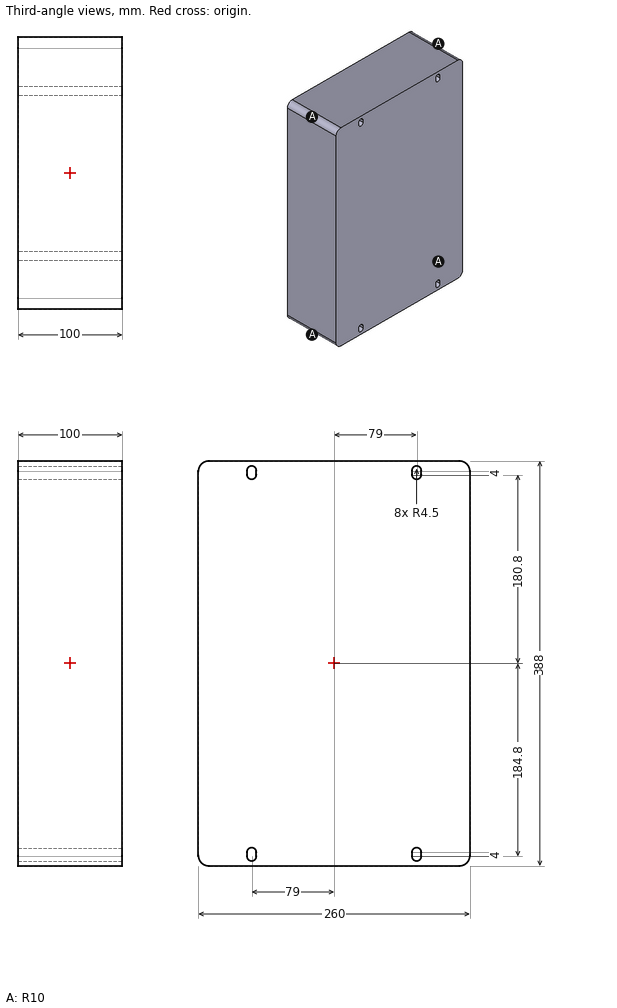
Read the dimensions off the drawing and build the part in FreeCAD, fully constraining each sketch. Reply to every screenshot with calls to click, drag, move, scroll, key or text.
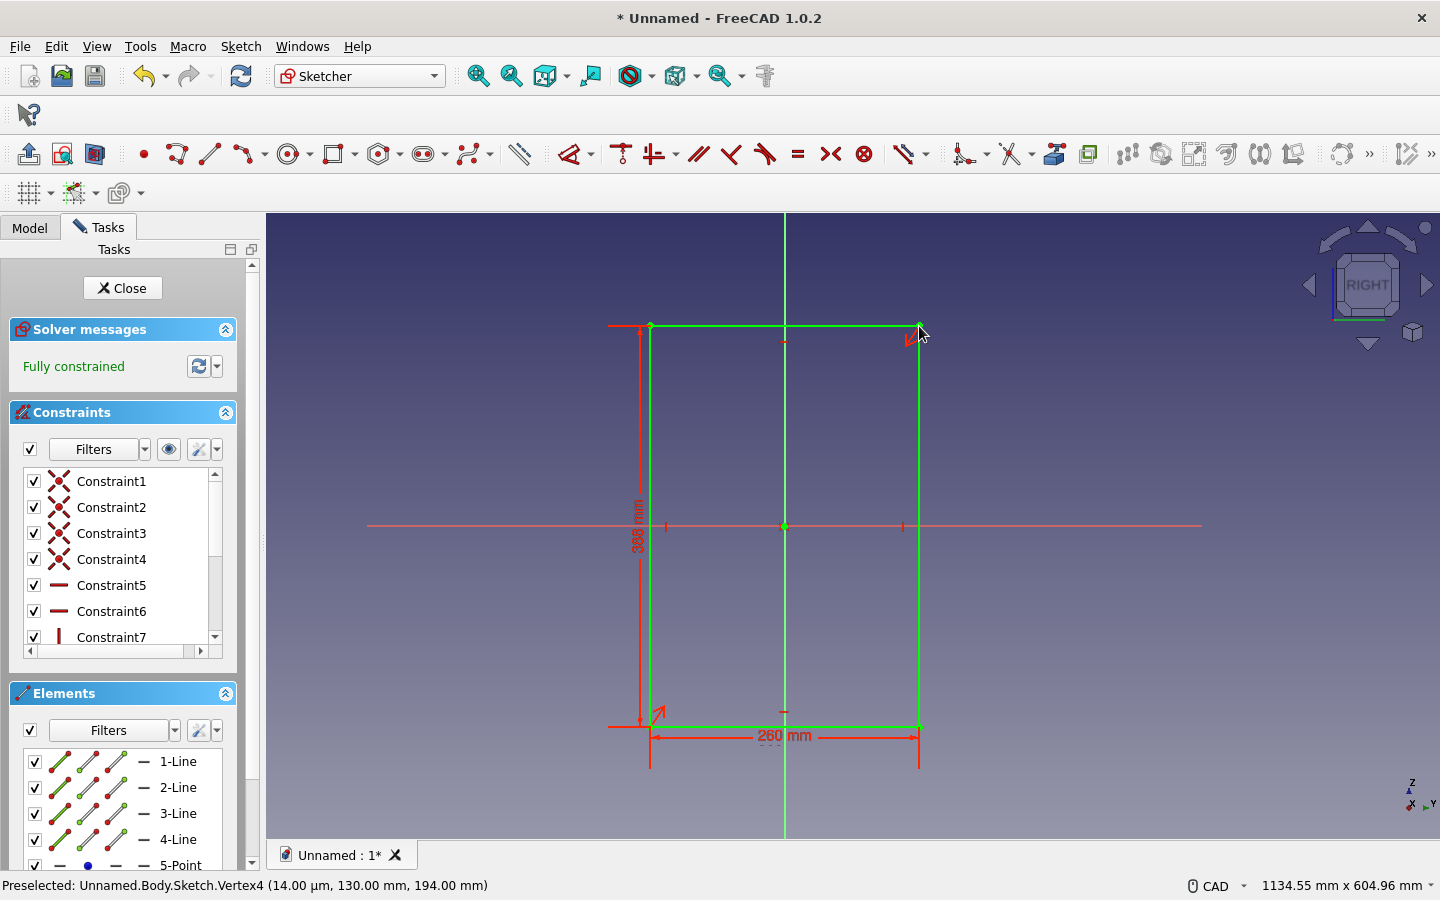
click(123, 288)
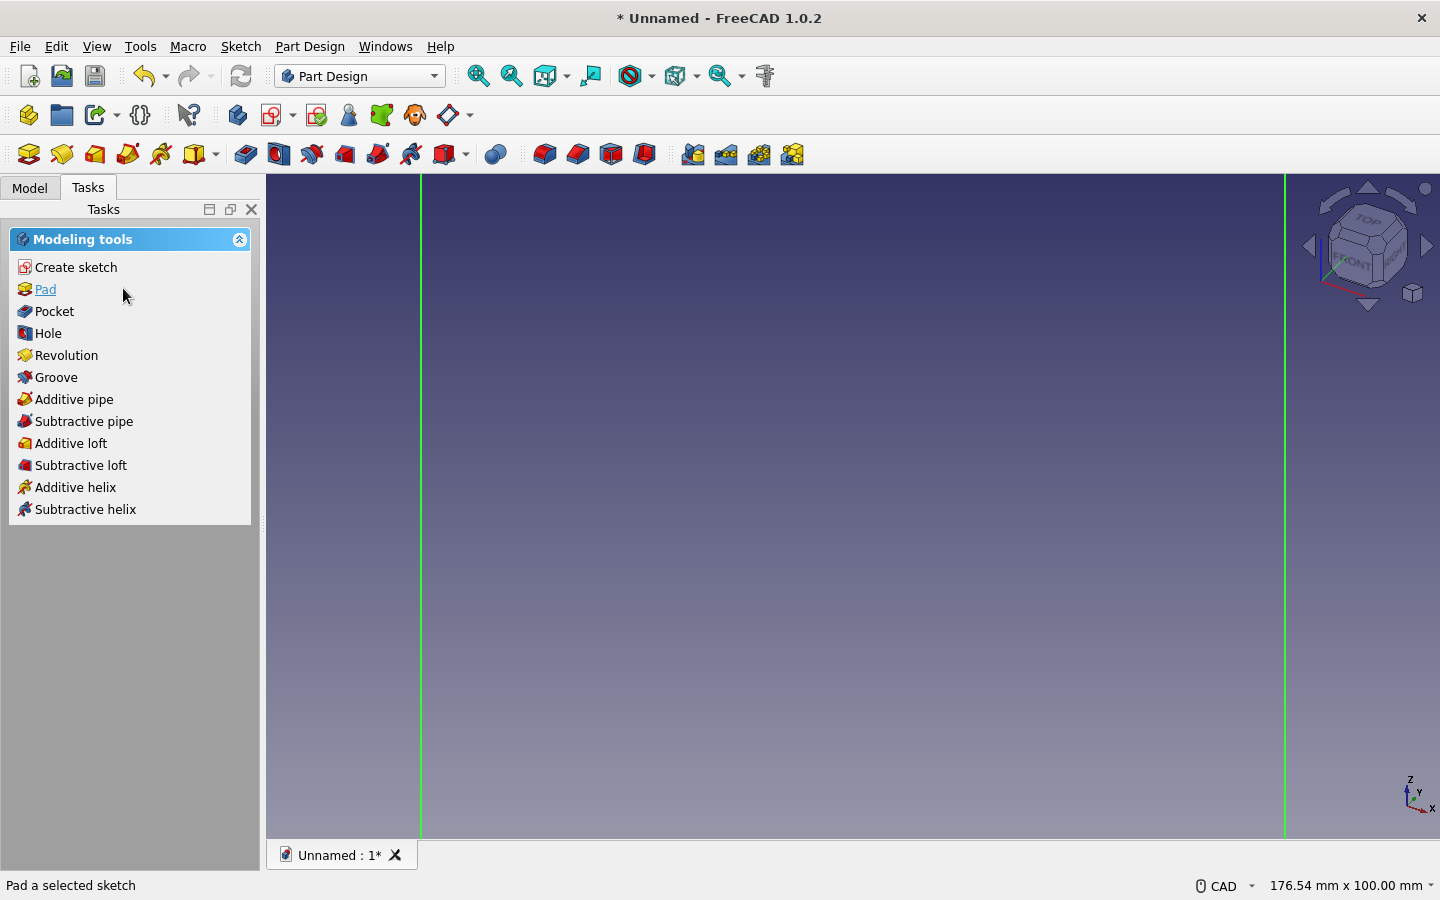
click(29, 154)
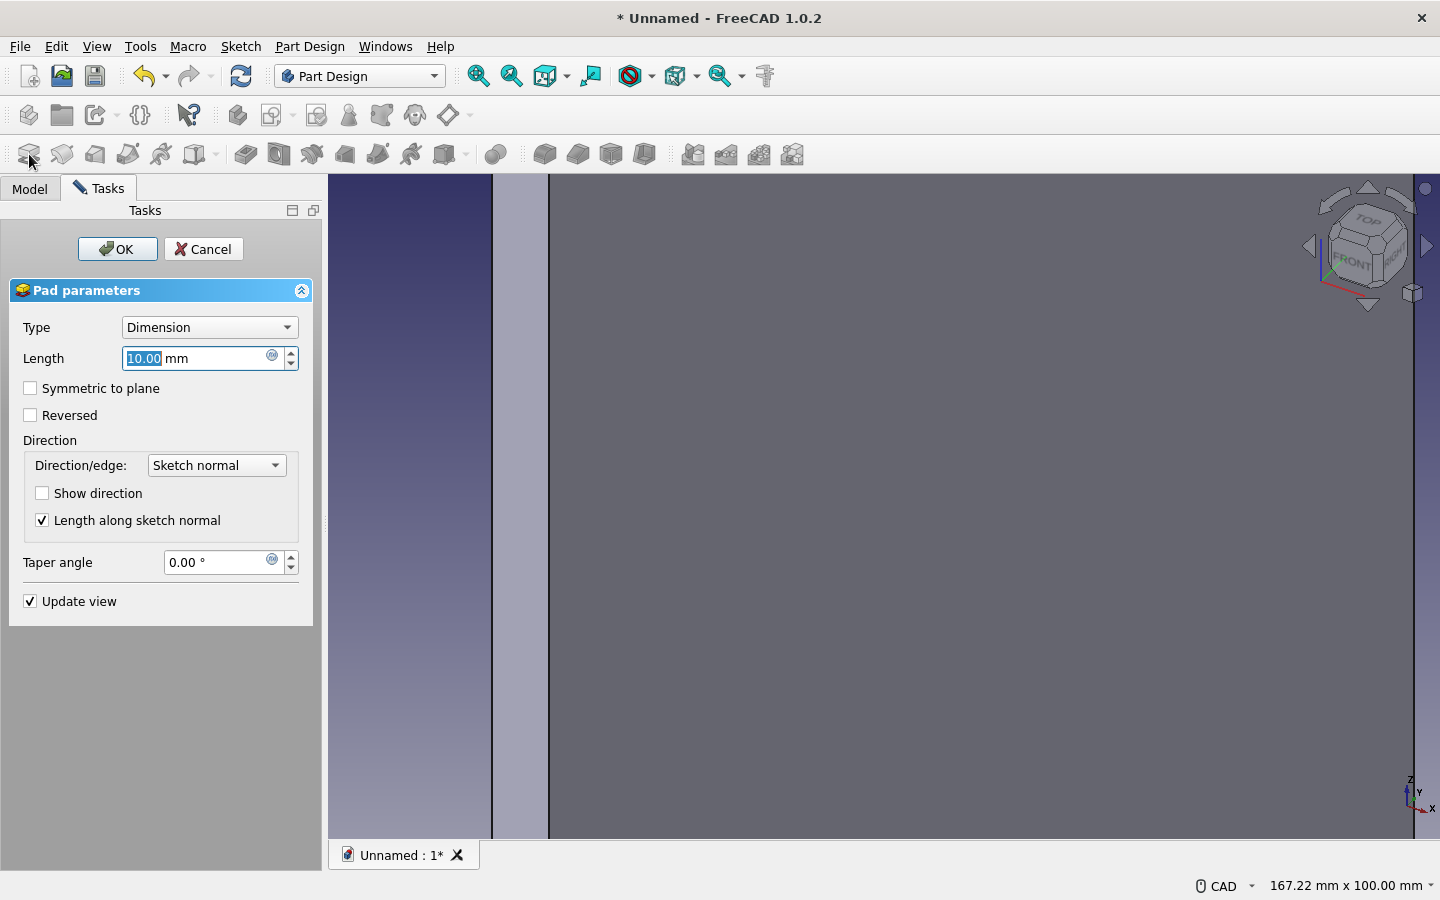
text(100)
key(Tab)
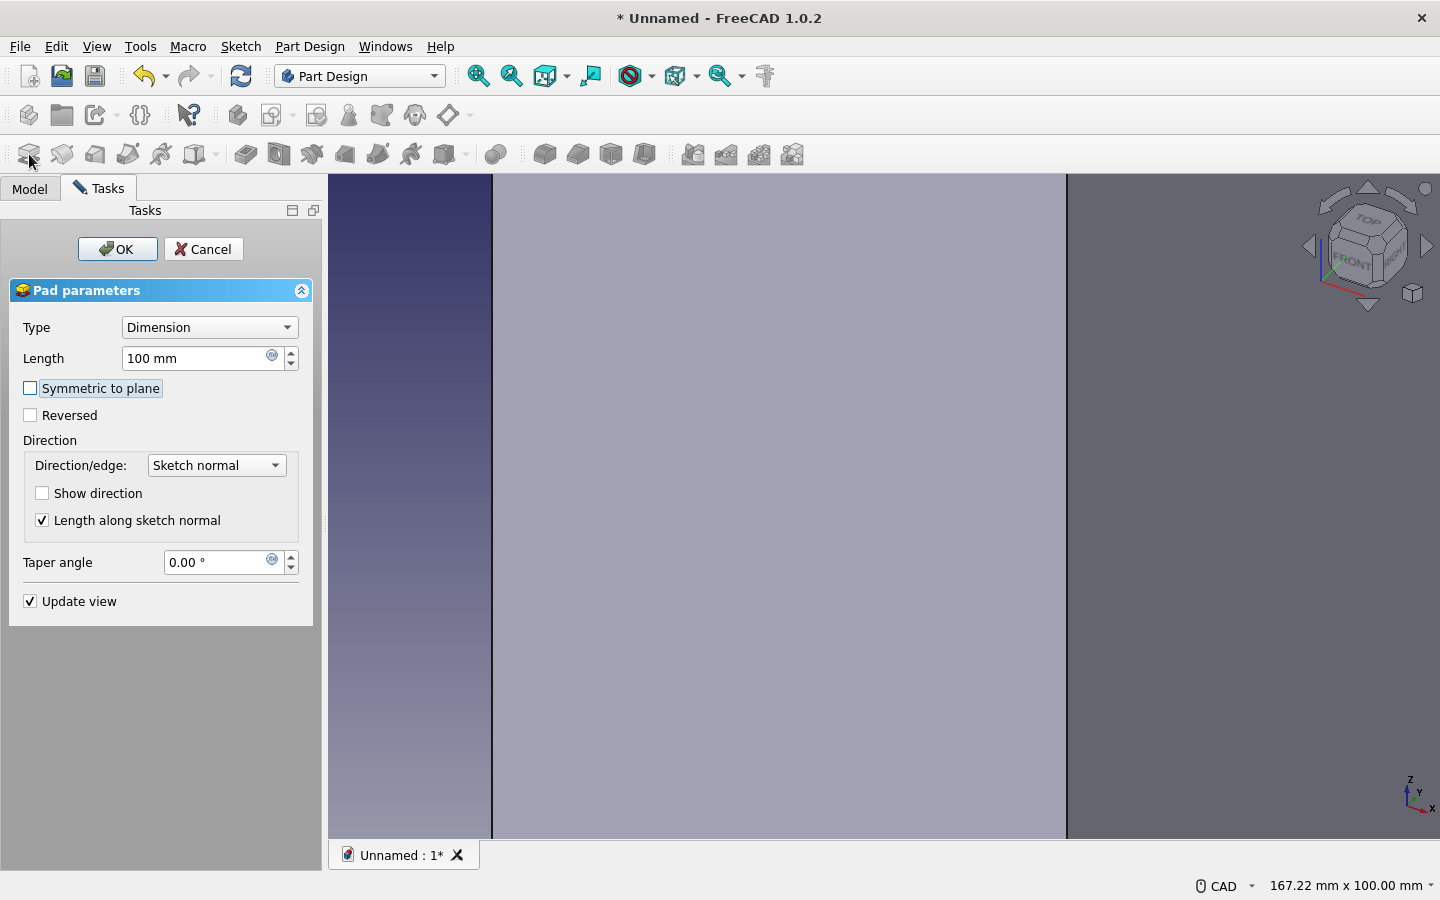
click(31, 388)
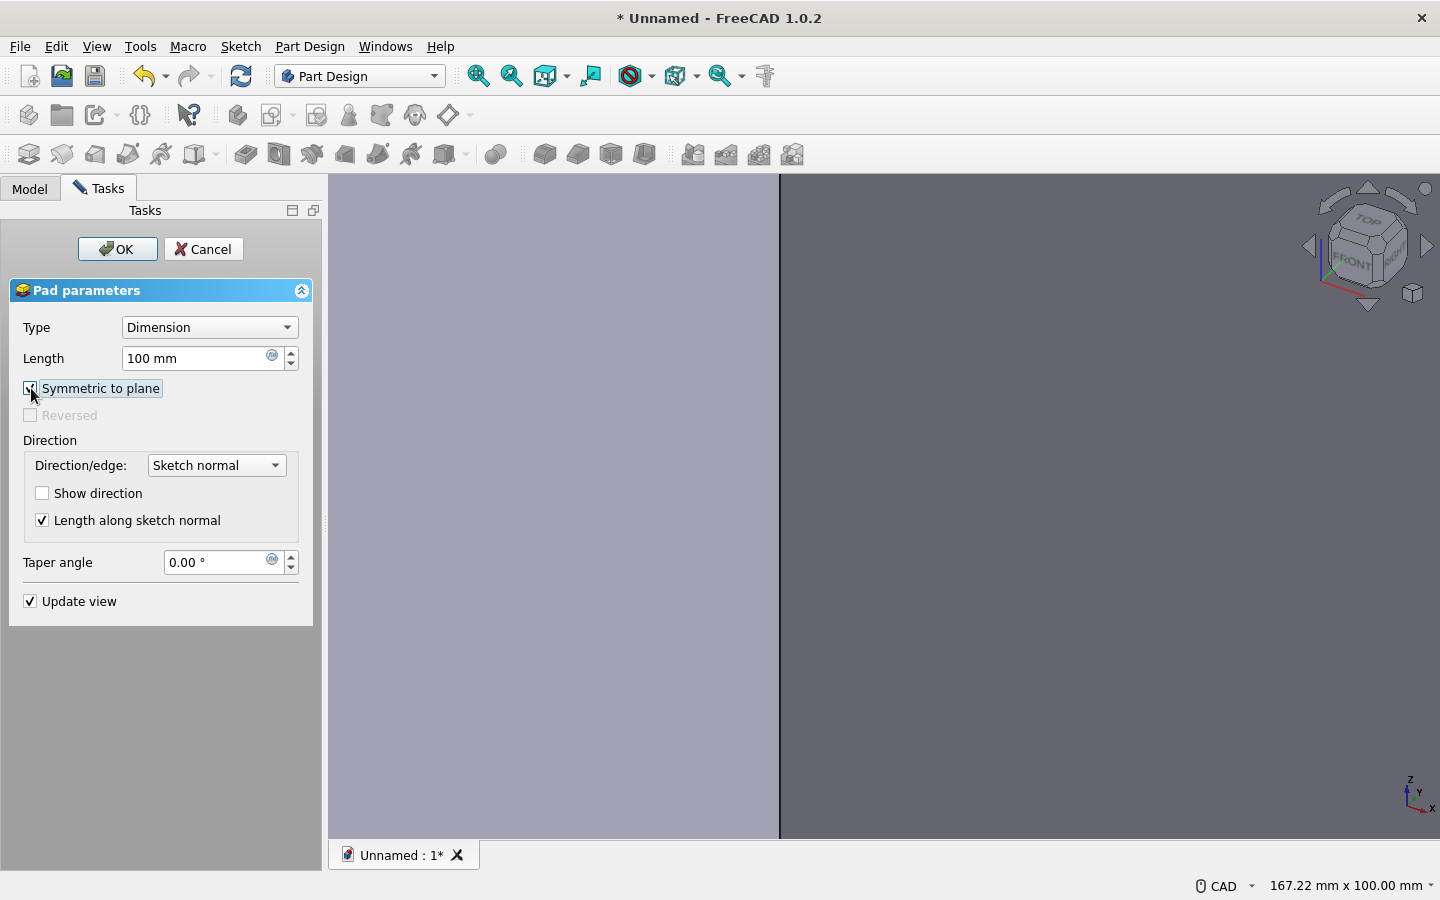
click(118, 249)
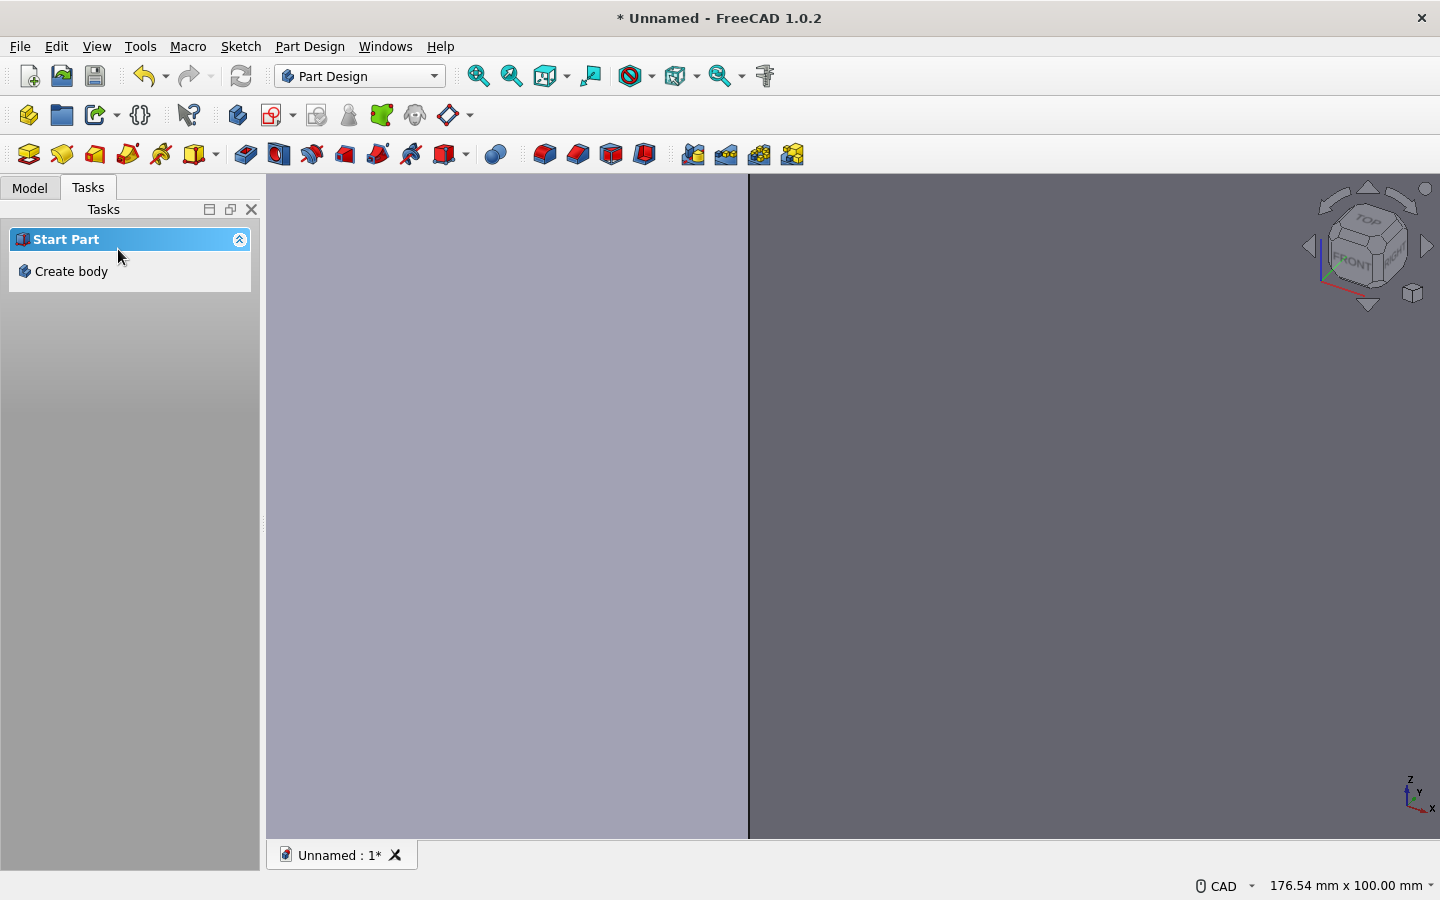
click(479, 76)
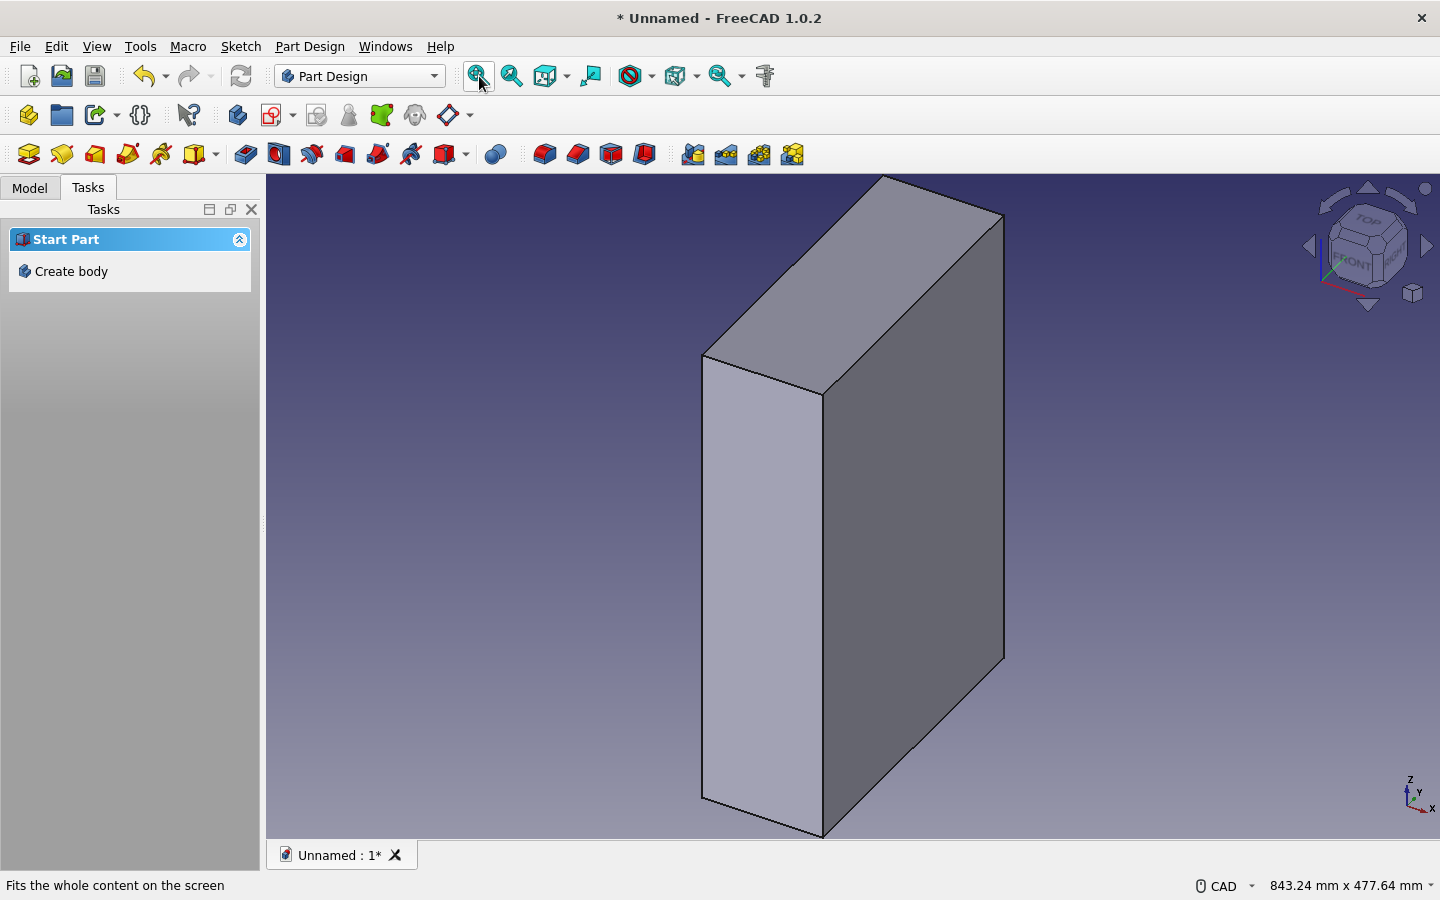
click(913, 525)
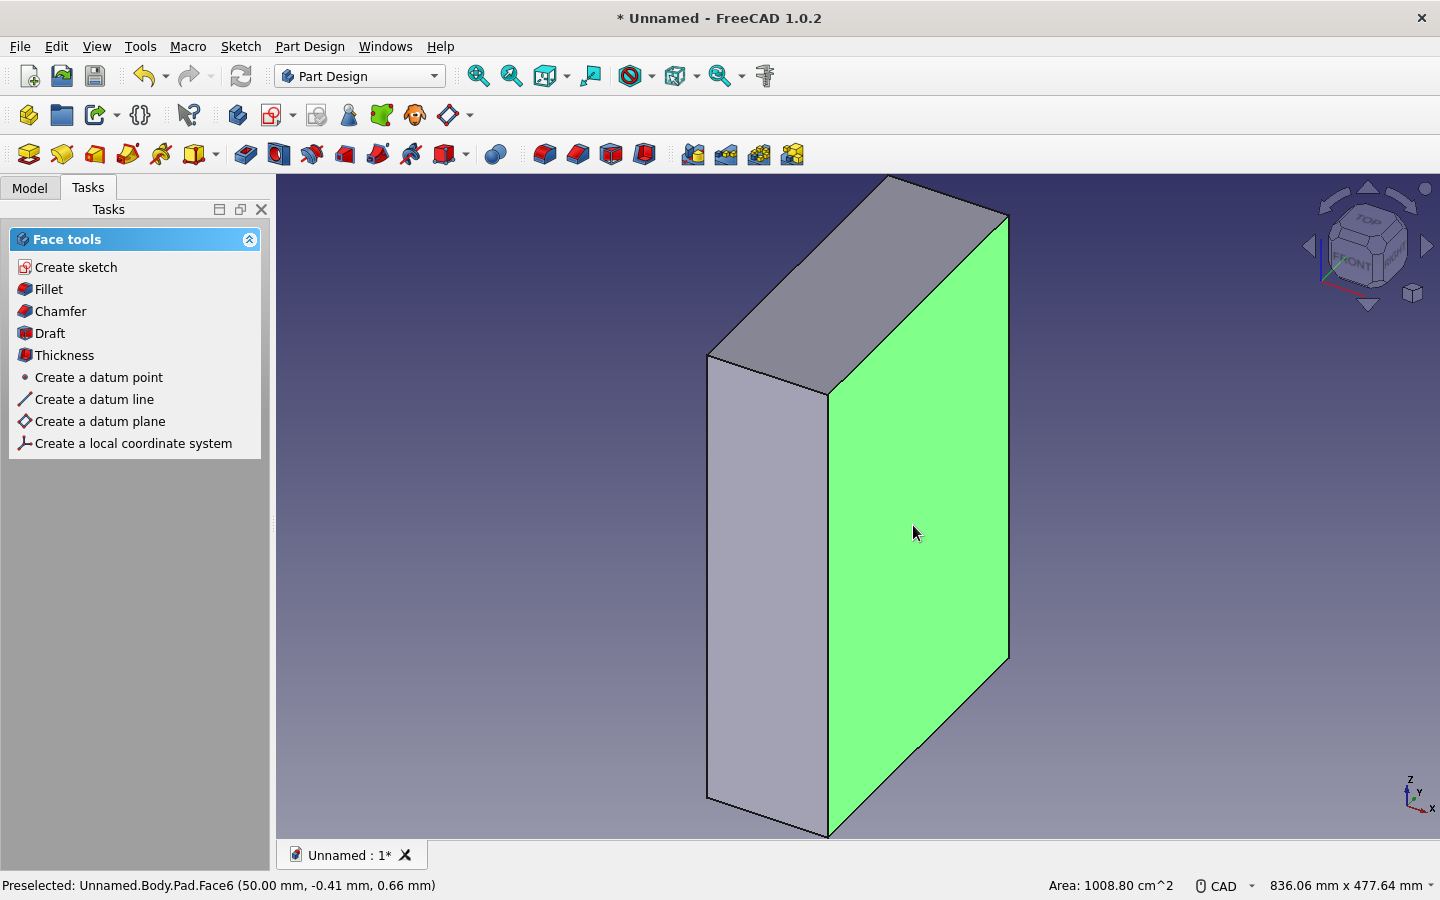
click(270, 116)